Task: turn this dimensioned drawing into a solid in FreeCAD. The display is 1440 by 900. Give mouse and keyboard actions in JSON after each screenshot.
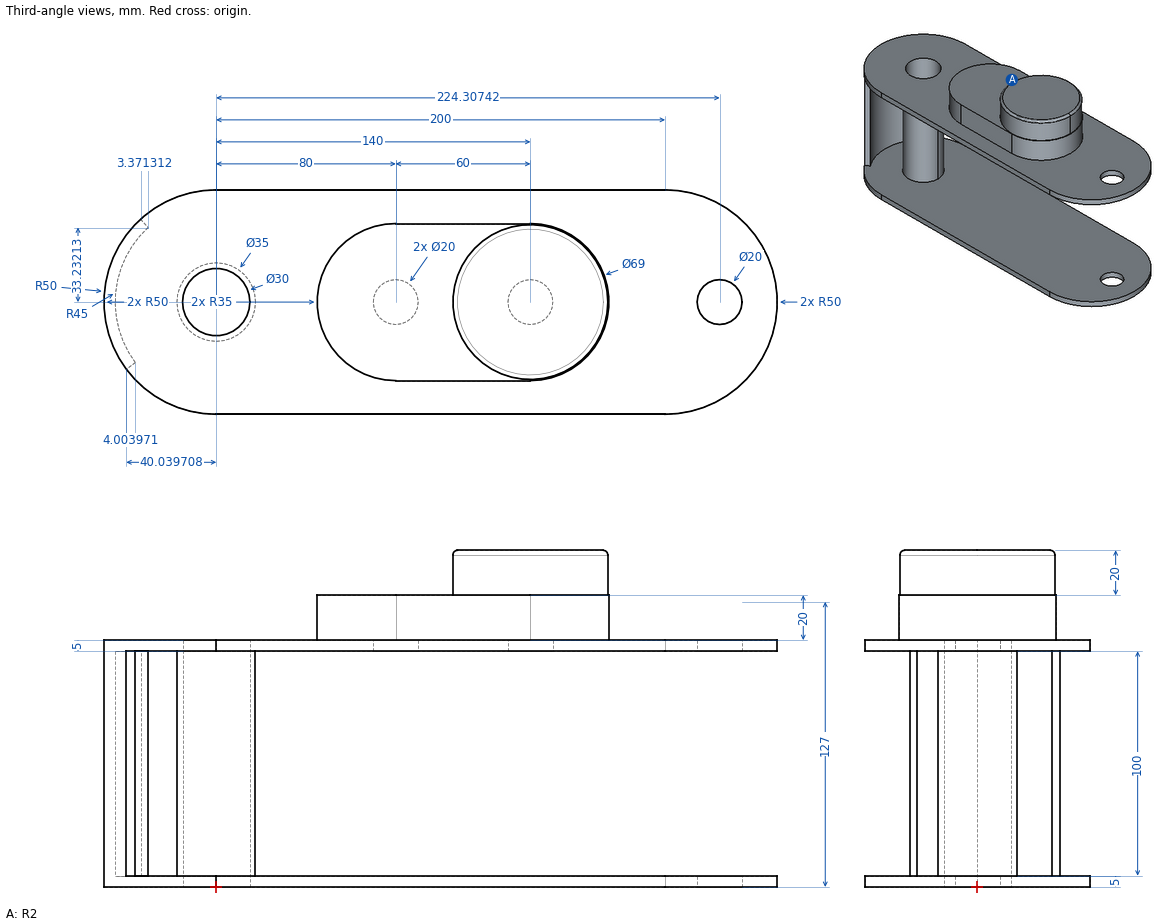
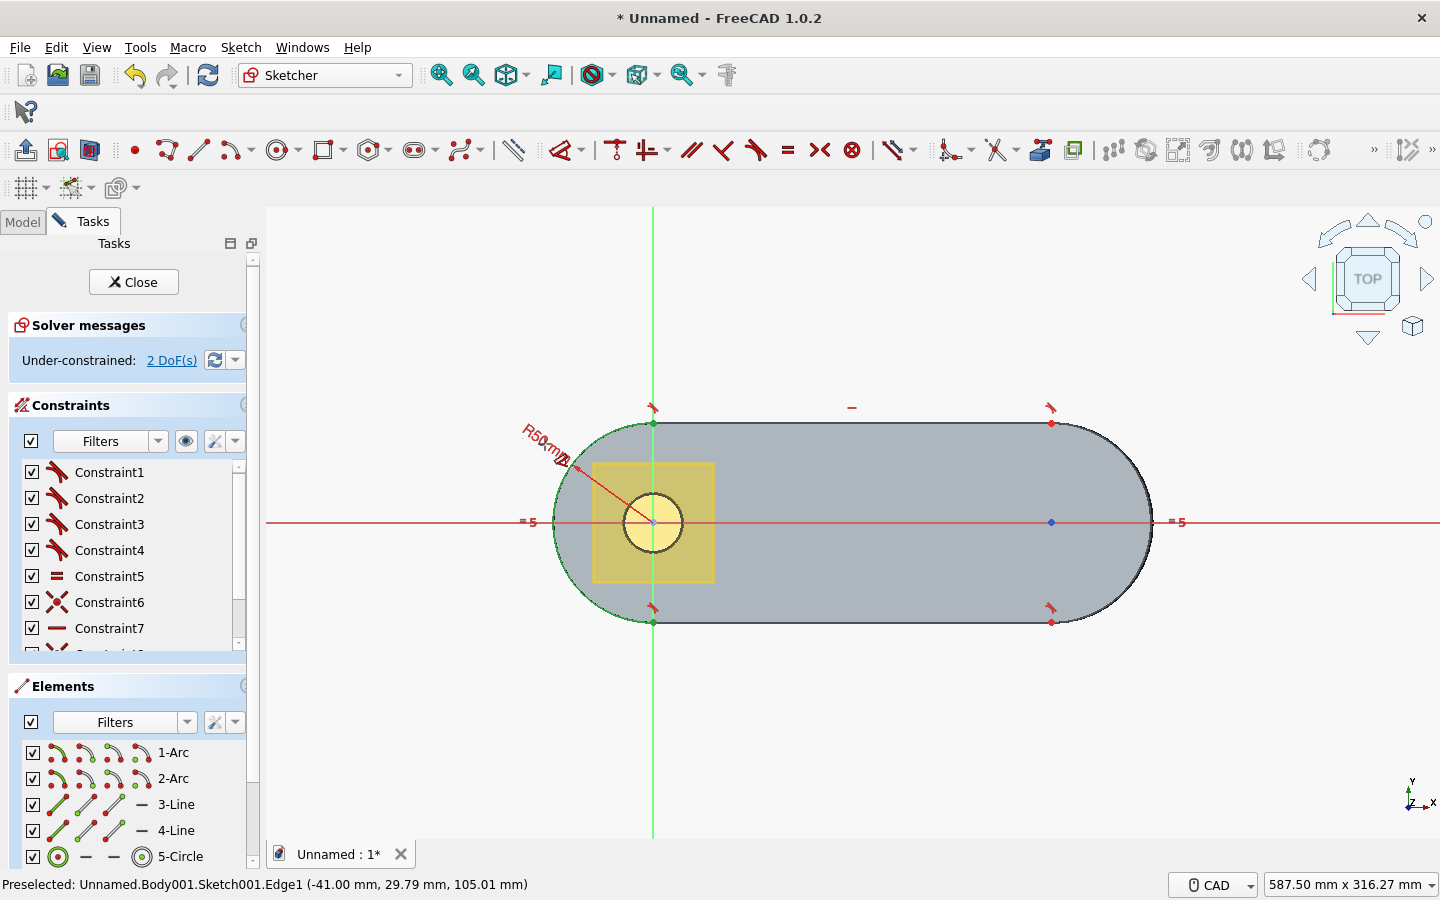
{"action": "left_click", "coordinate": [674, 503]}
{"action": "left_click", "coordinate": [697, 481]}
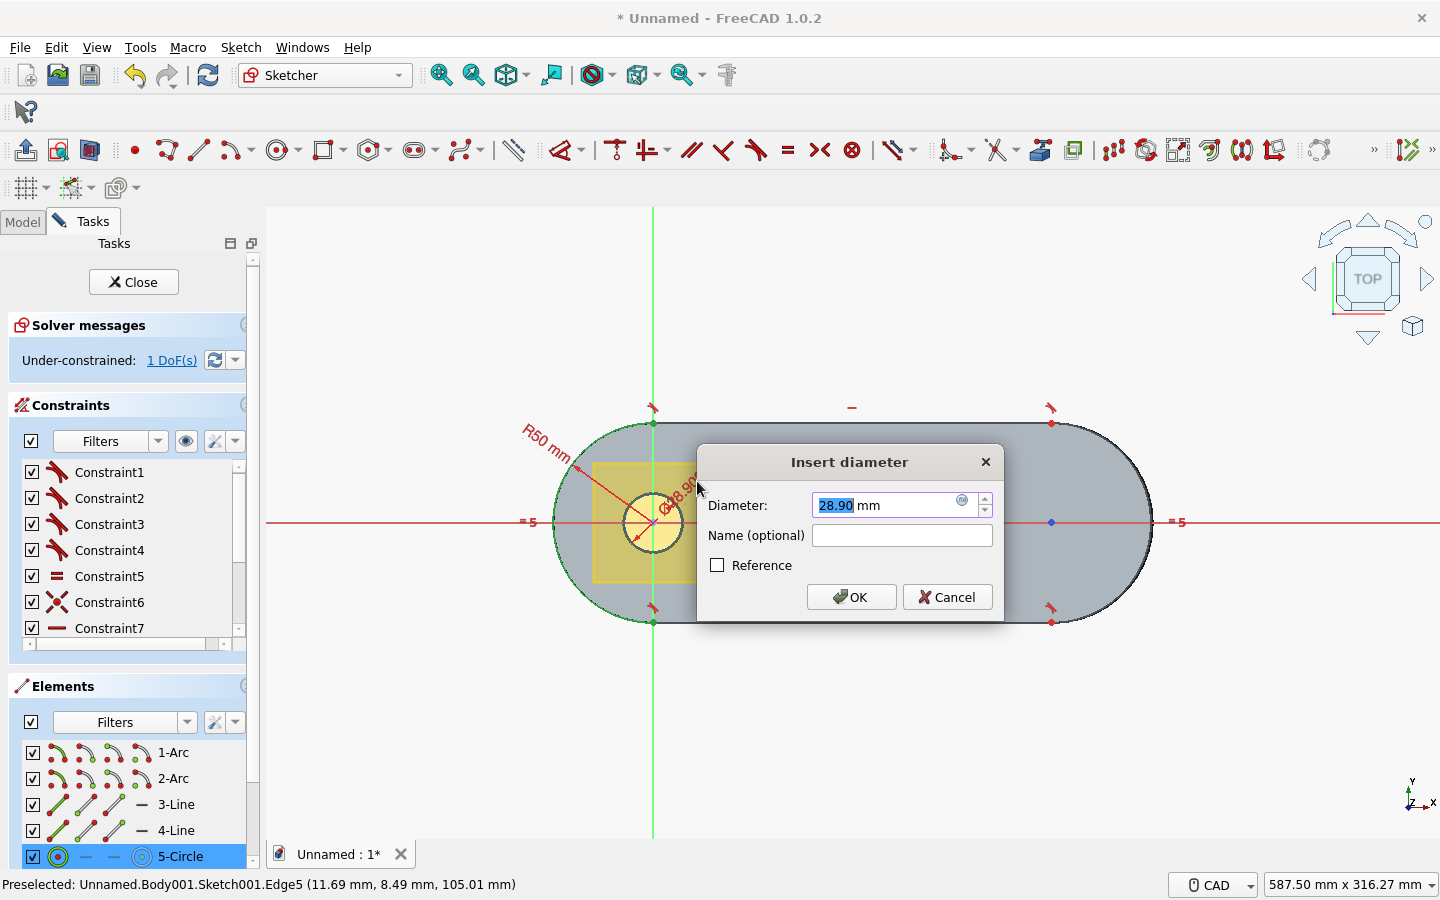
{"action": "type", "text": "30"}
{"action": "key", "text": "Return"}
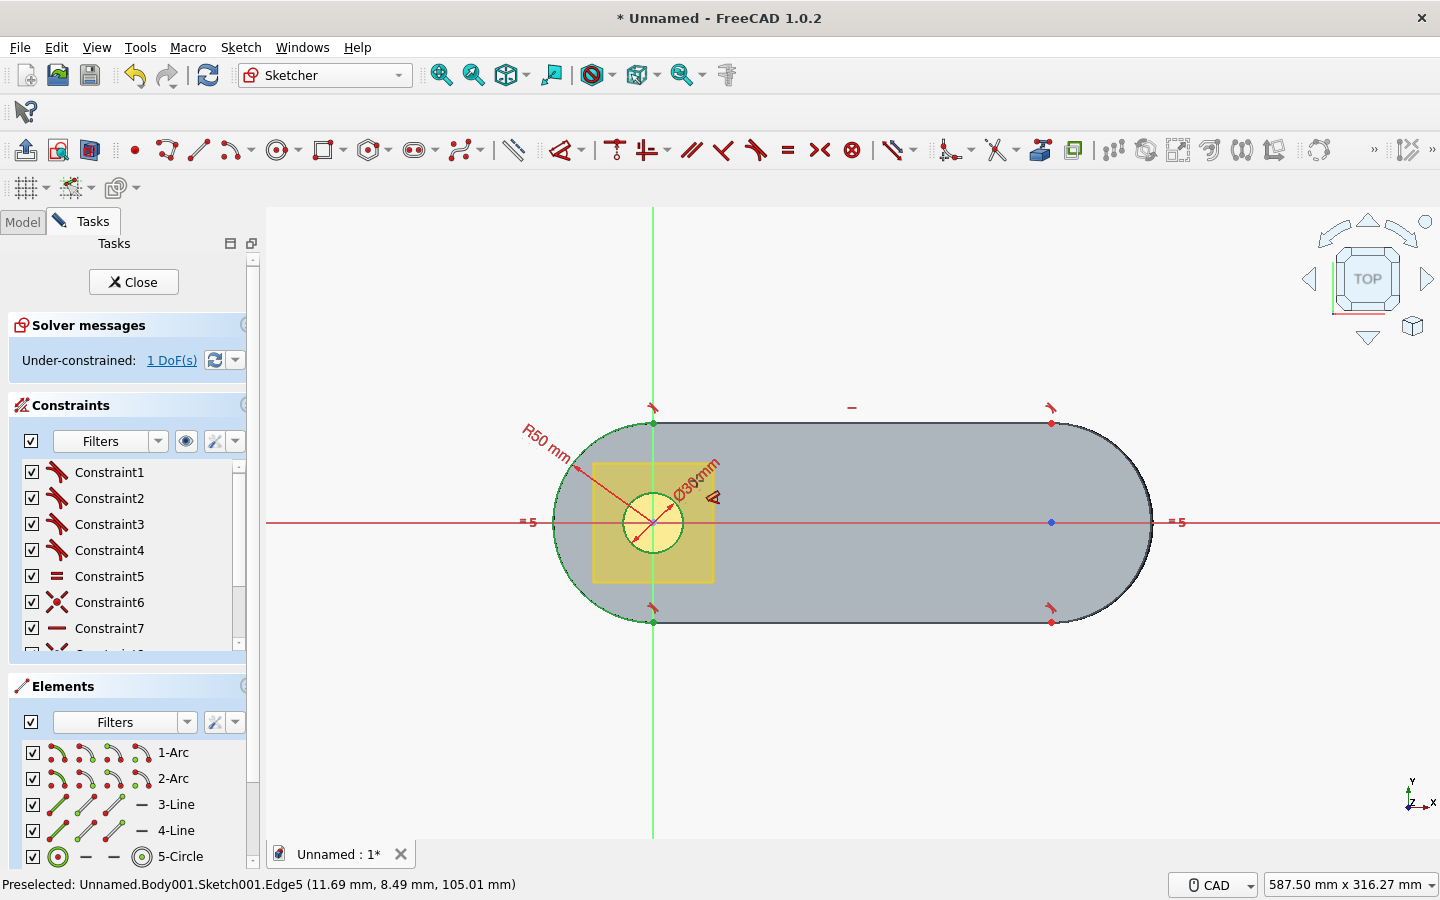
{"action": "left_click", "coordinate": [773, 423]}
{"action": "left_click", "coordinate": [852, 389]}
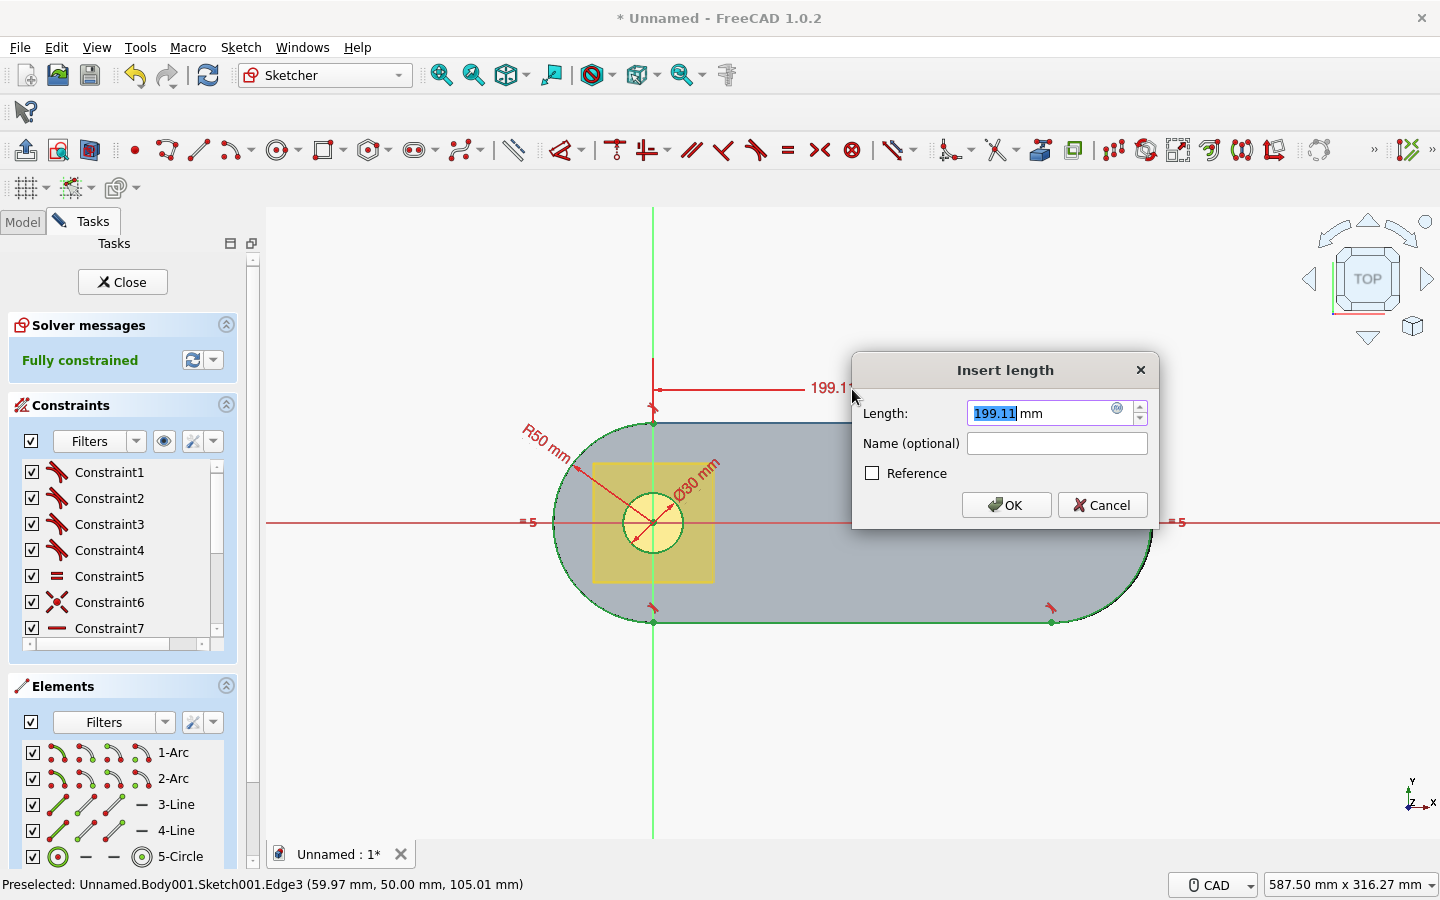
{"action": "type", "text": "200"}
{"action": "key", "text": "Return"}
{"action": "key", "text": "Escape"}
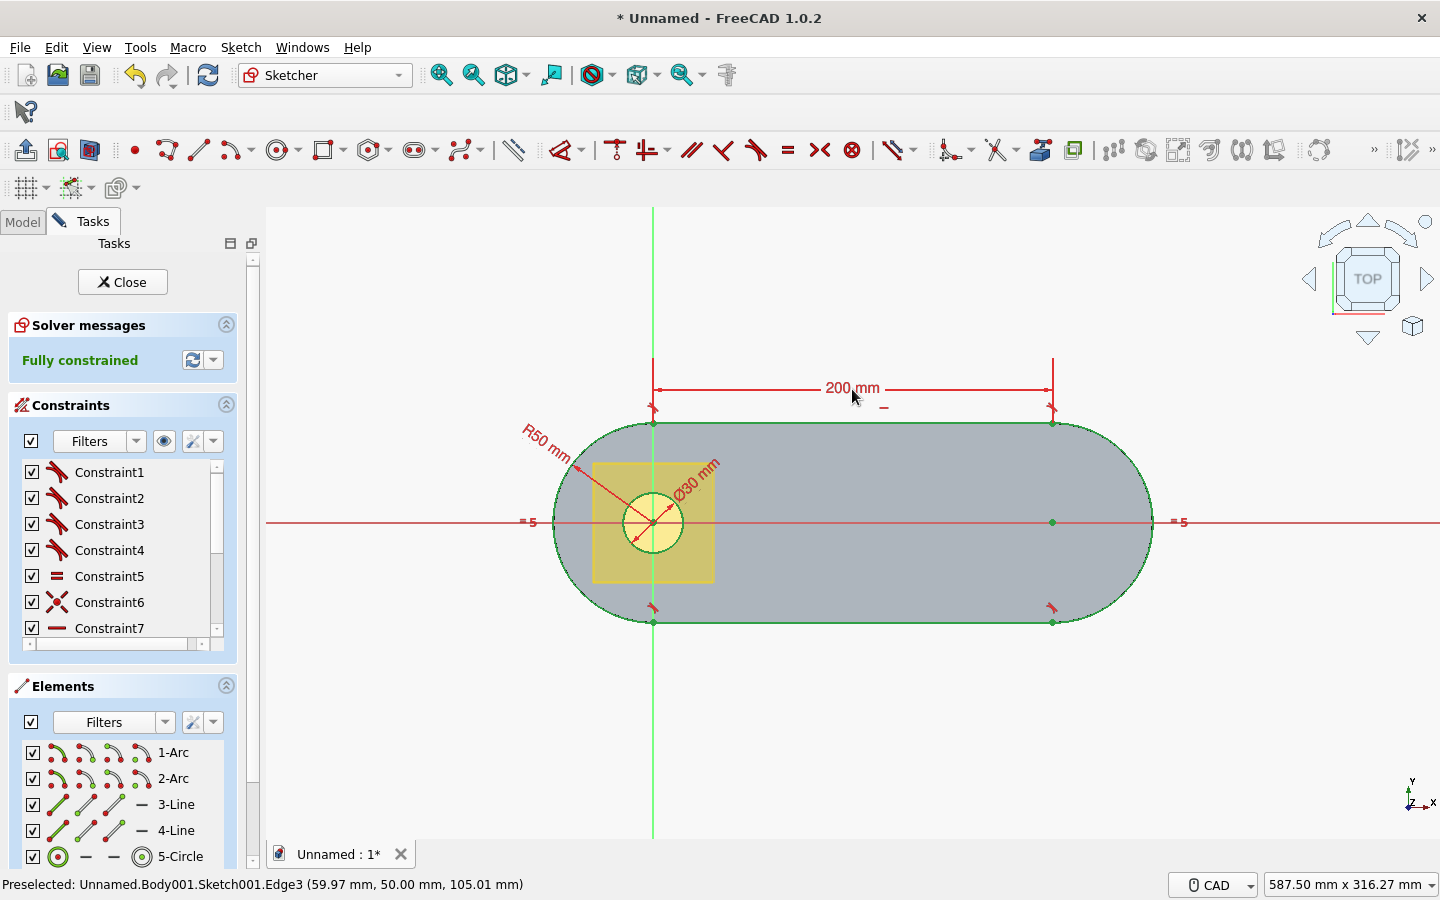
{"action": "left_click", "coordinate": [123, 282]}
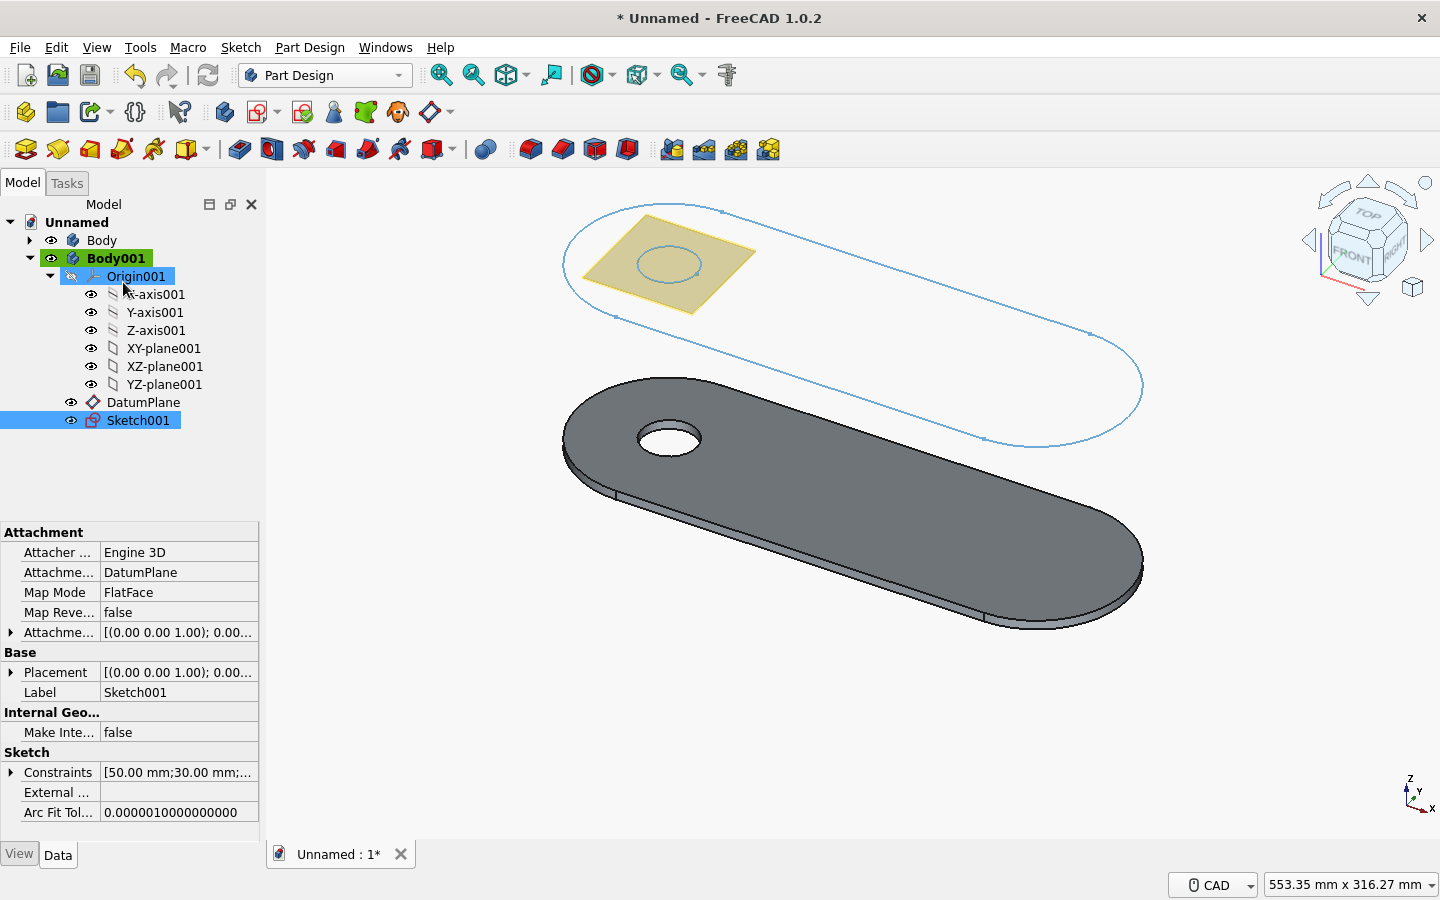
{"action": "left_click", "coordinate": [26, 150]}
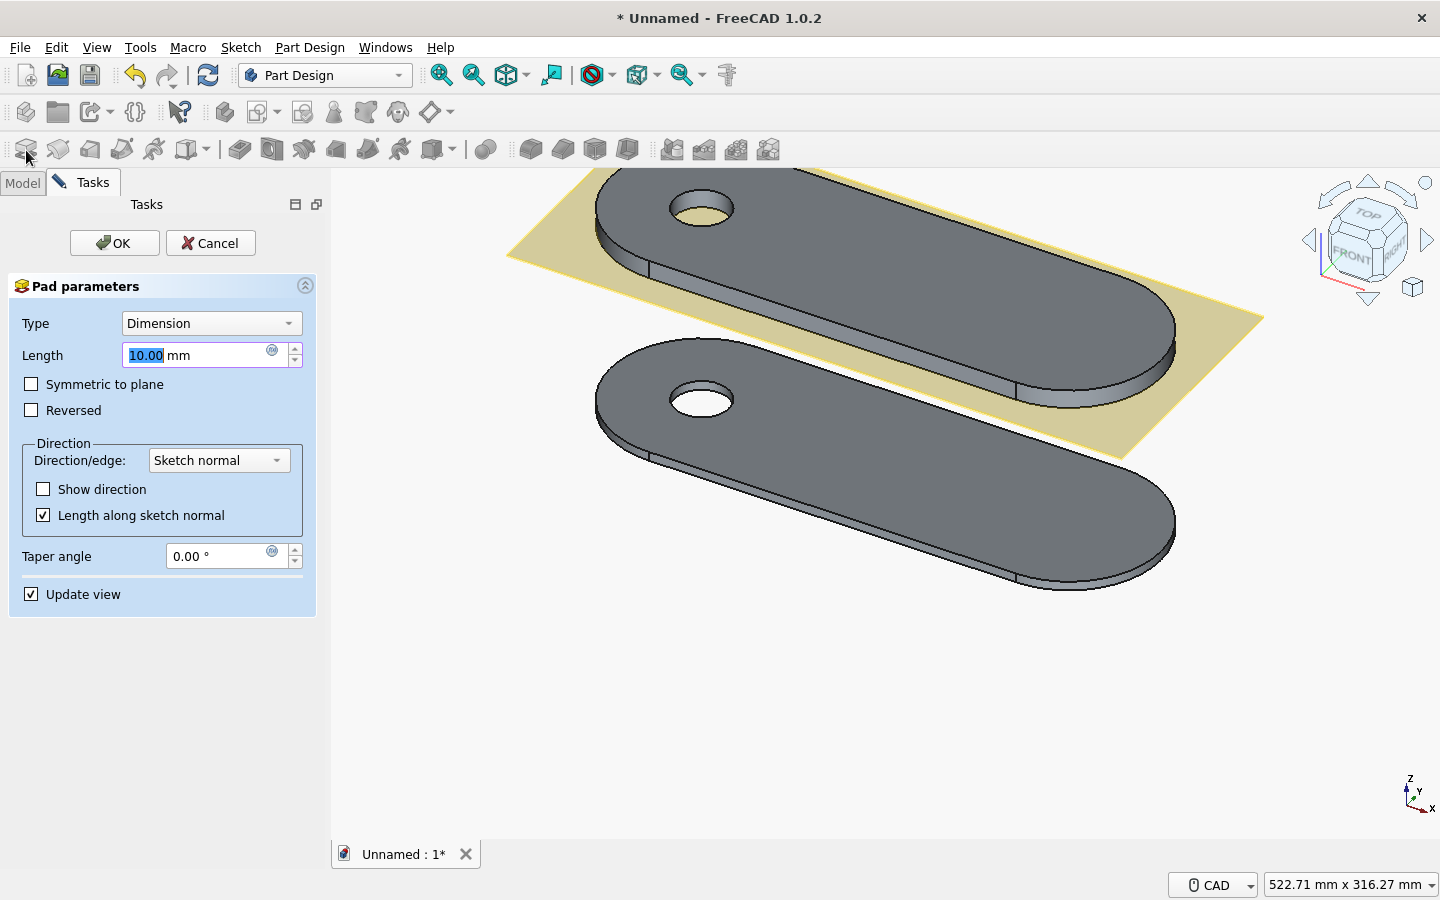
{"action": "type", "text": "5"}
{"action": "key", "text": "Tab"}